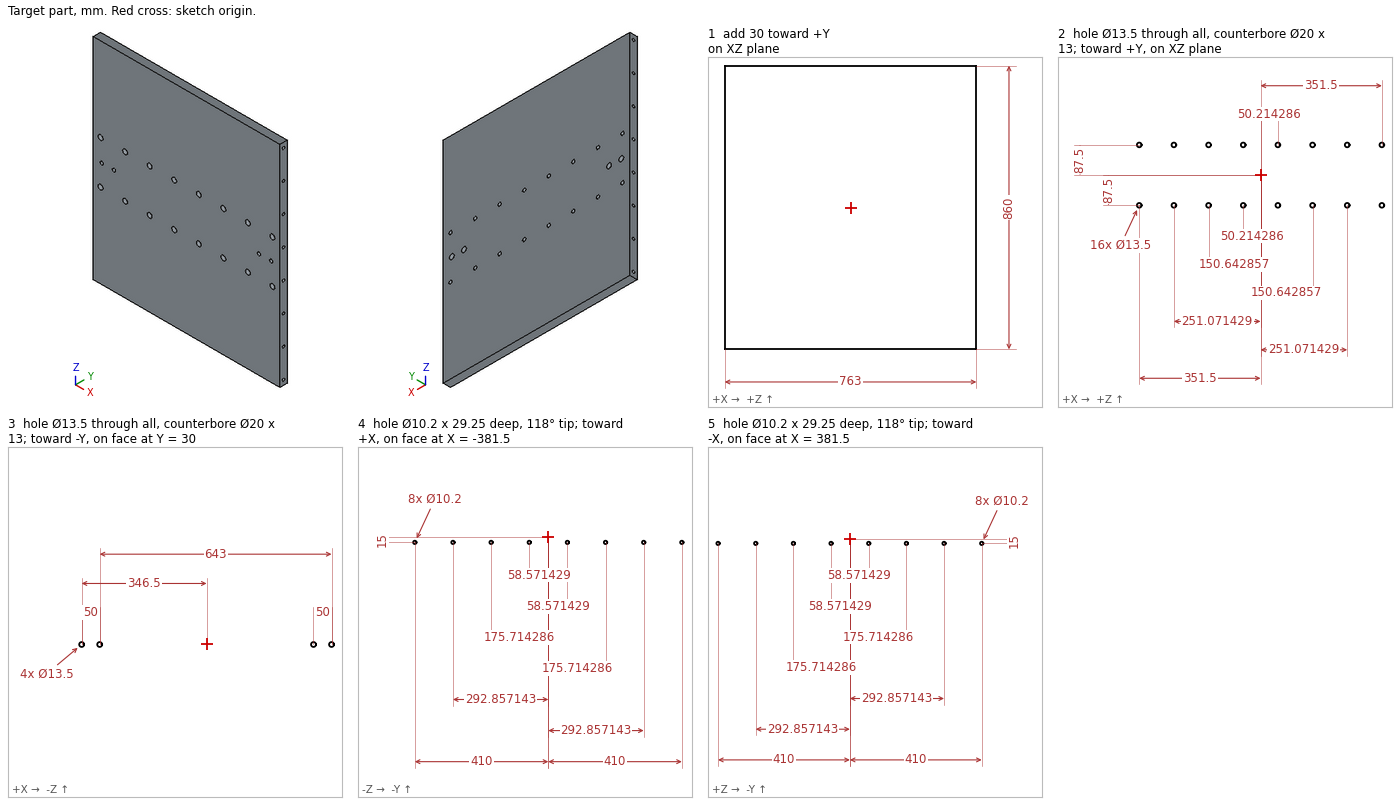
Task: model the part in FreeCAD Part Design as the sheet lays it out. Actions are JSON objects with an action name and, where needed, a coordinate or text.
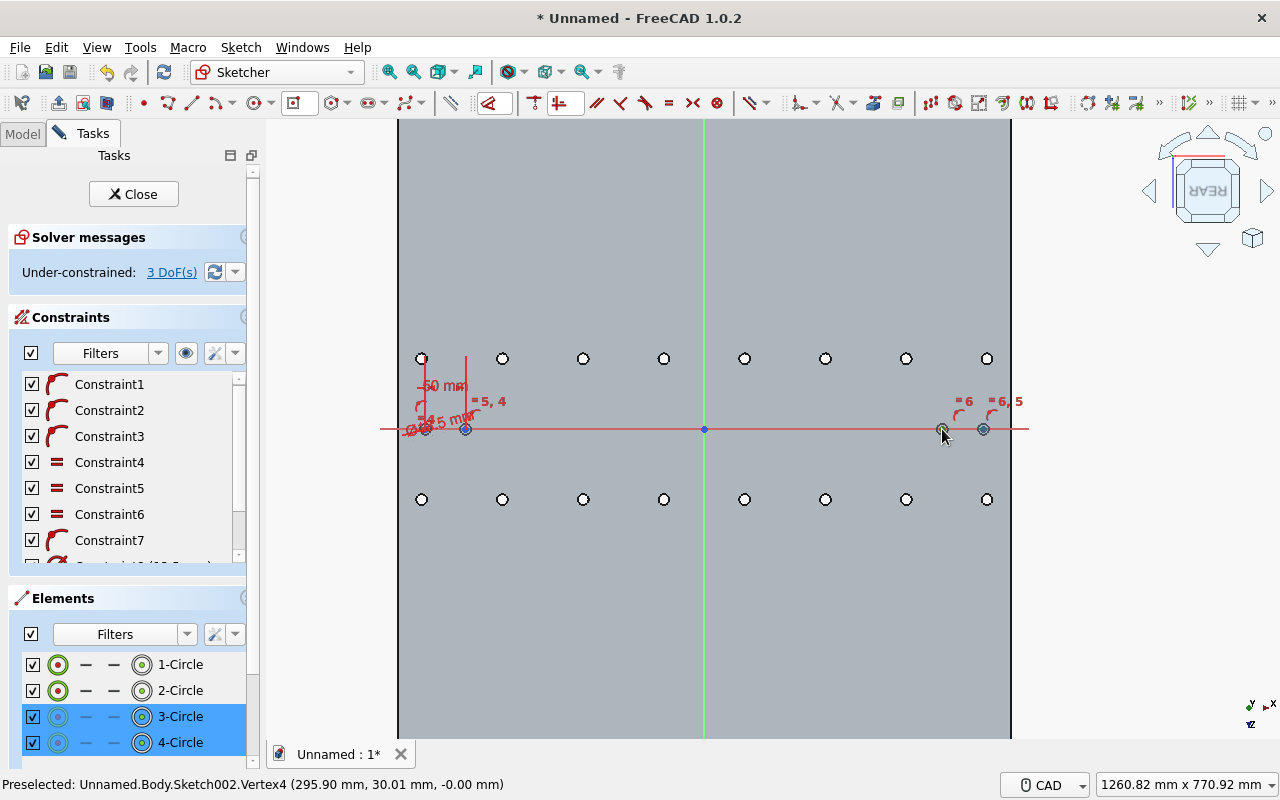
{"action": "key", "text": "l"}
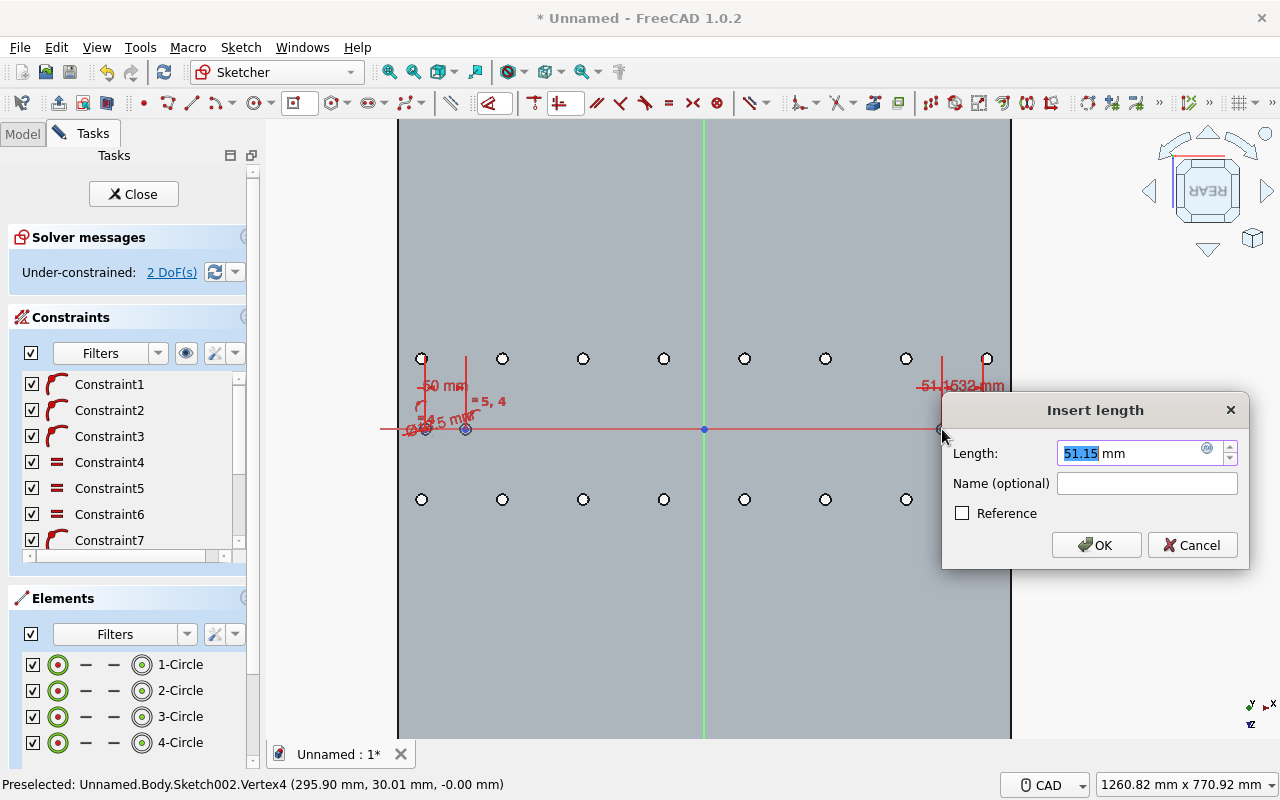
{"action": "type", "text": "50"}
{"action": "key", "text": "Return"}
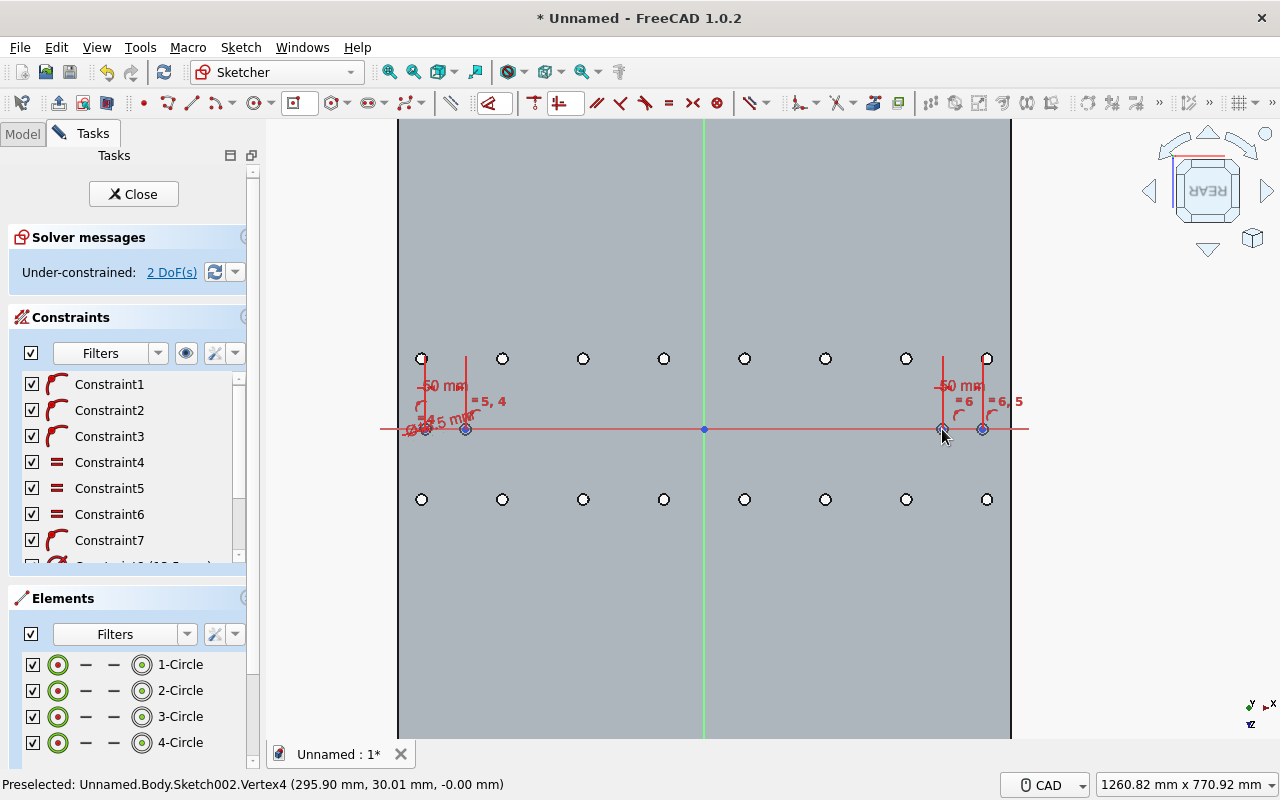
{"action": "left_click", "coordinate": [466, 429]}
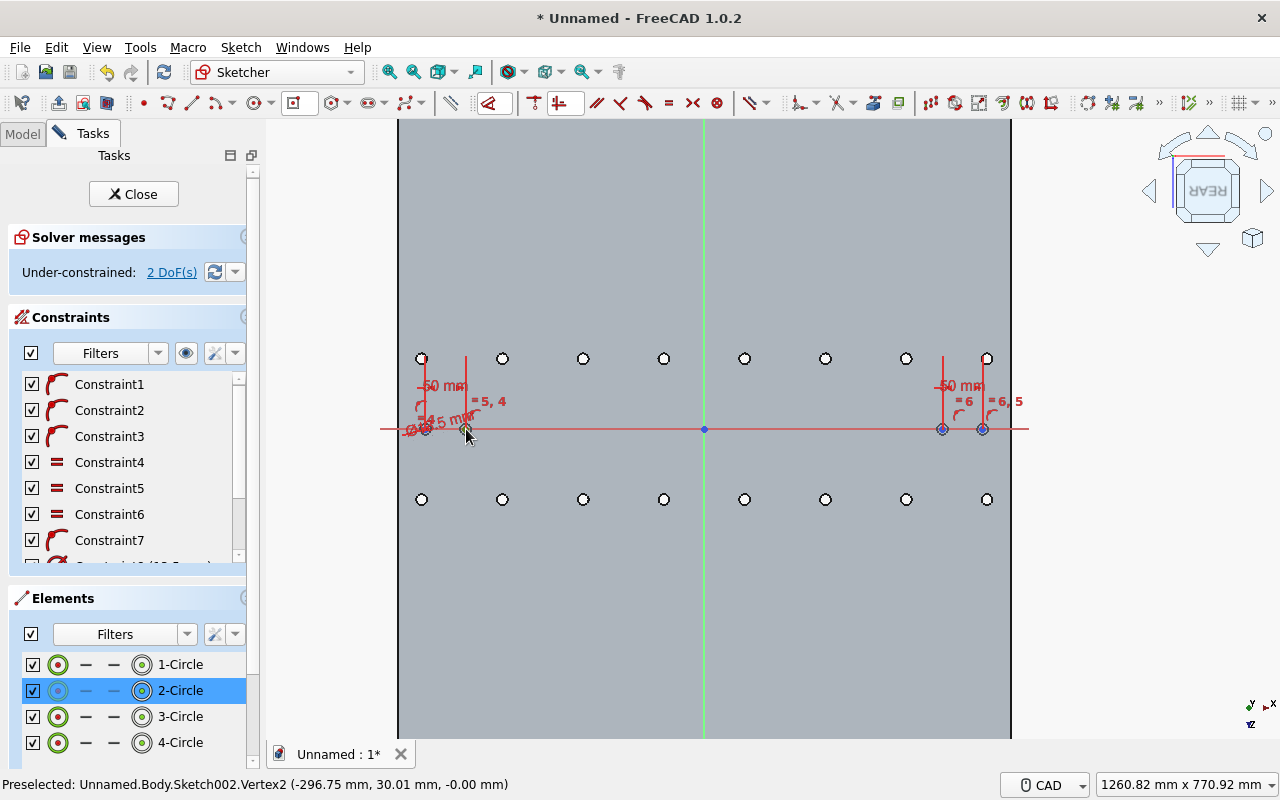
{"action": "left_click", "coordinate": [983, 429]}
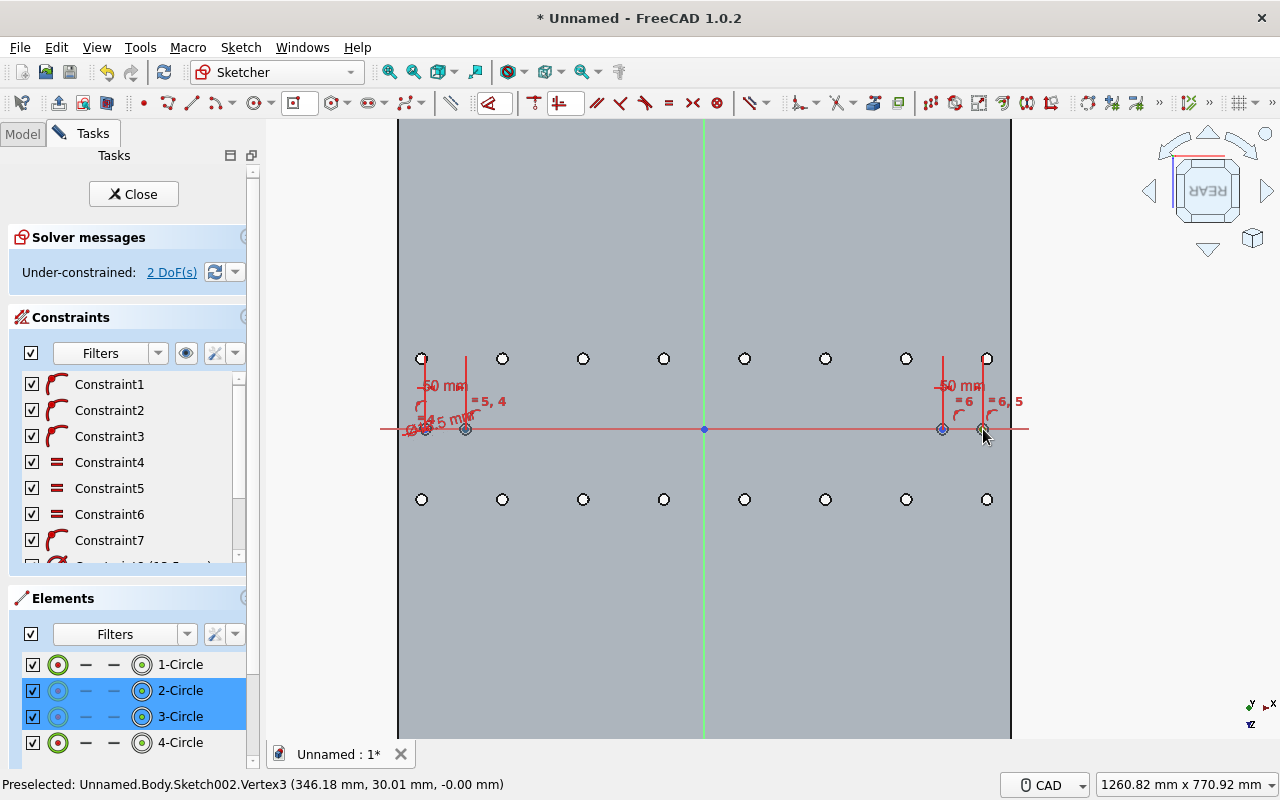
{"action": "key", "text": "l"}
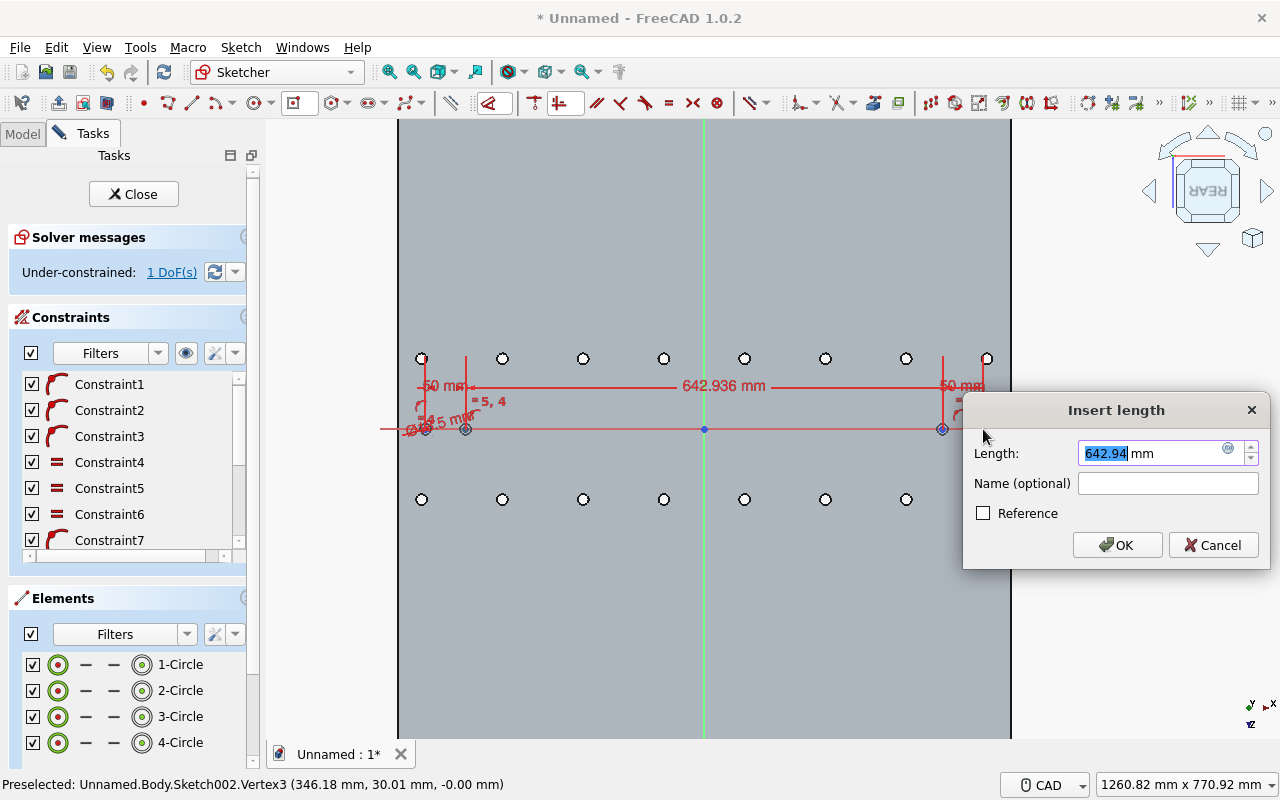
{"action": "type", "text": "643"}
{"action": "key", "text": "Return"}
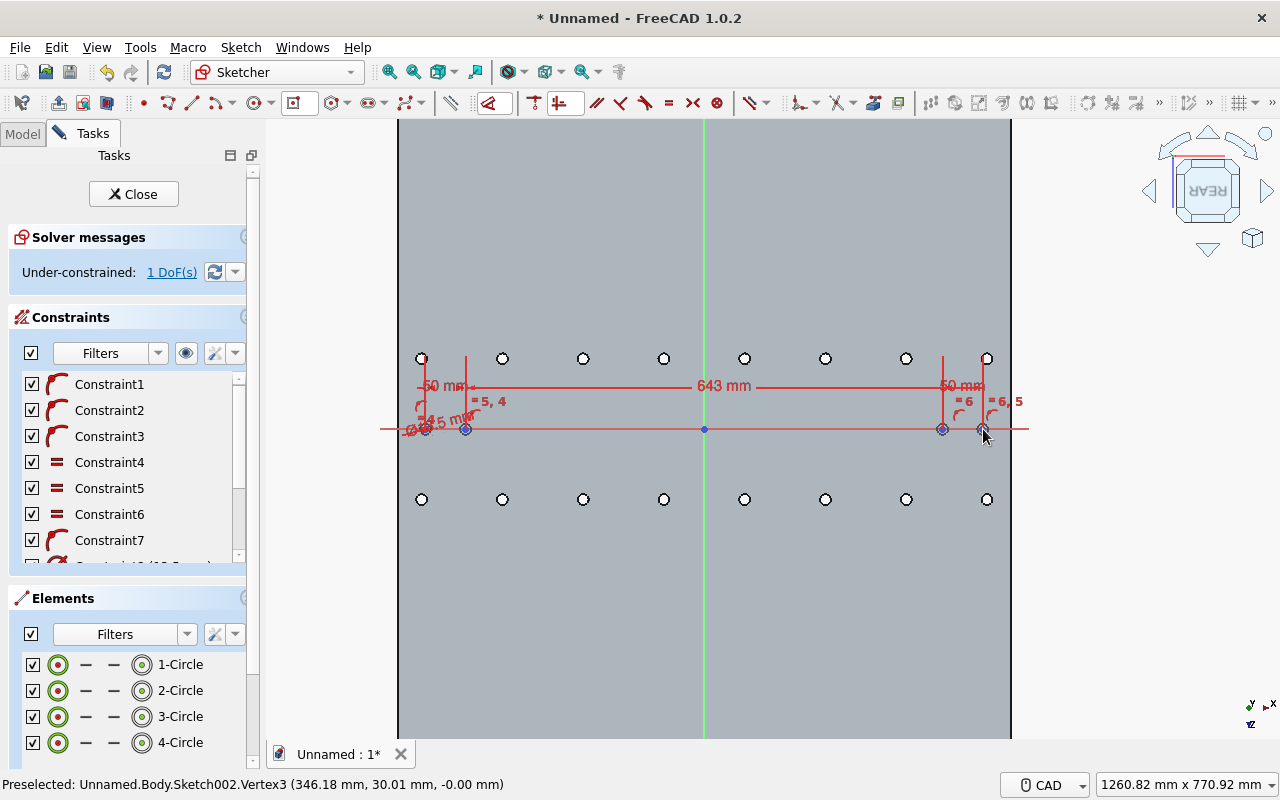
{"action": "left_click", "coordinate": [425, 429]}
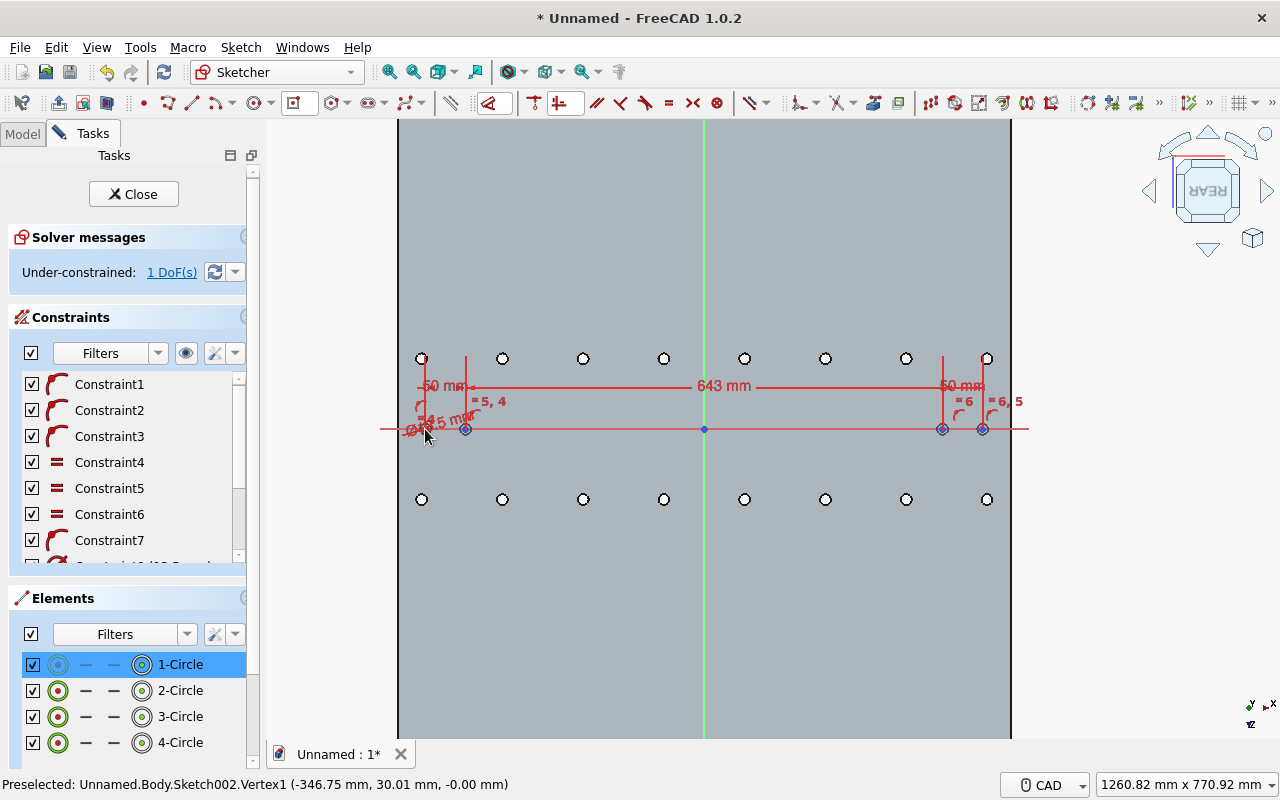
{"action": "left_click", "coordinate": [506, 104]}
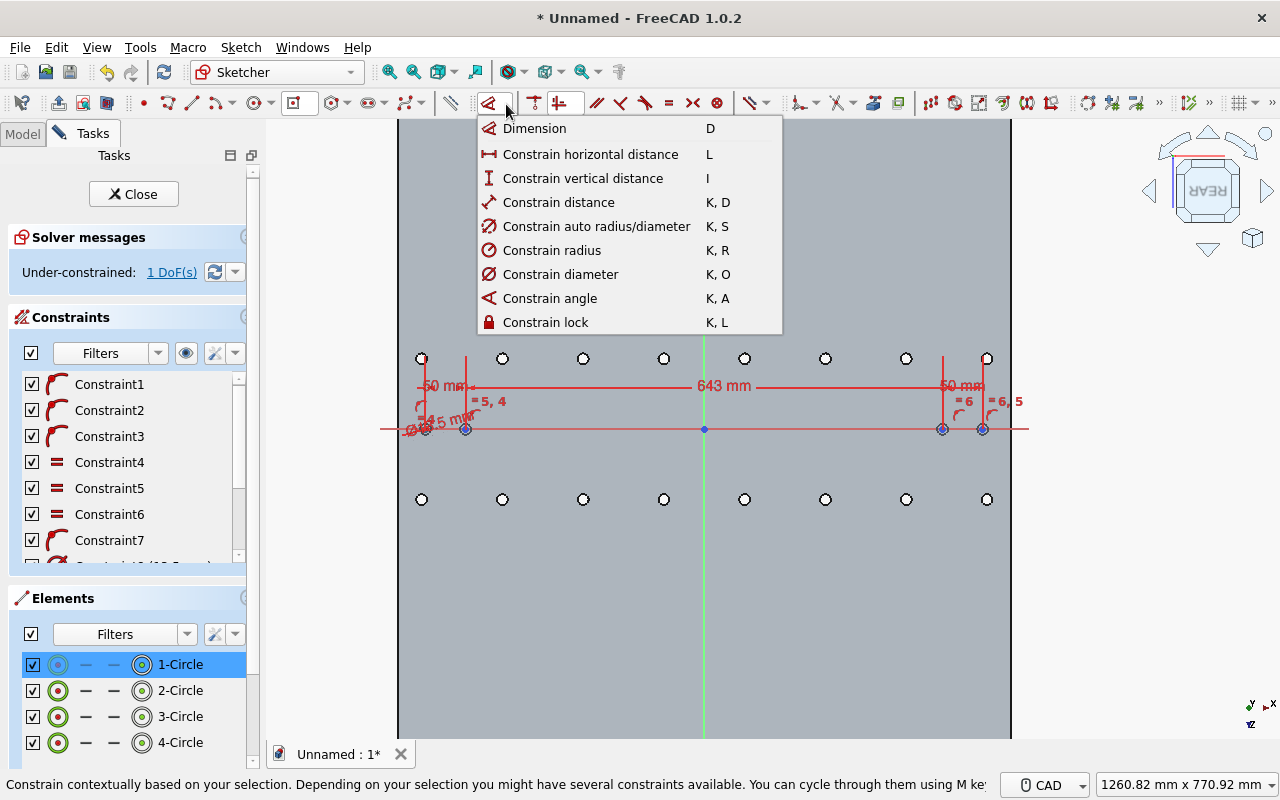
{"action": "left_click", "coordinate": [630, 154]}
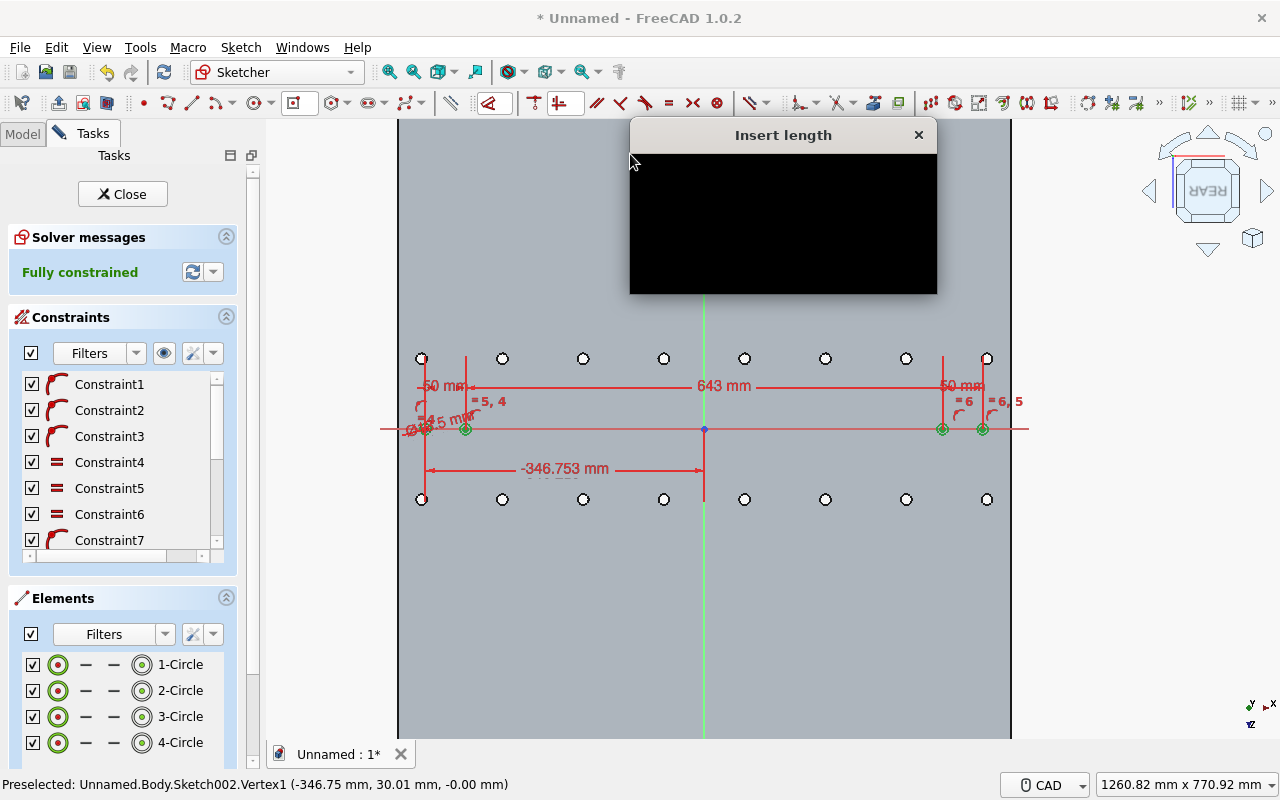
{"action": "type", "text": "-346.5"}
{"action": "key", "text": "Return"}